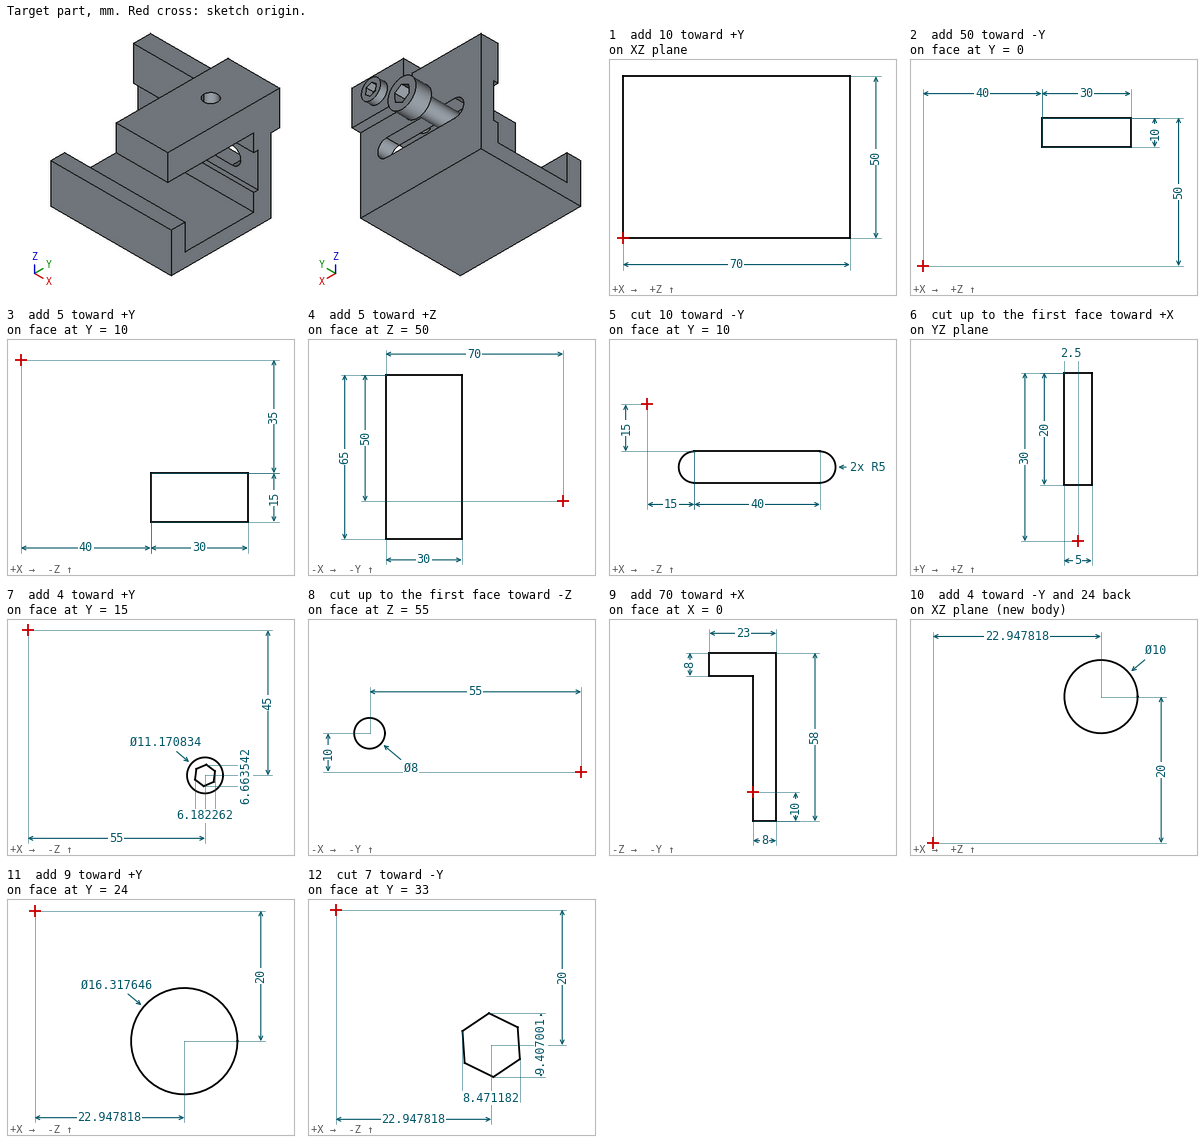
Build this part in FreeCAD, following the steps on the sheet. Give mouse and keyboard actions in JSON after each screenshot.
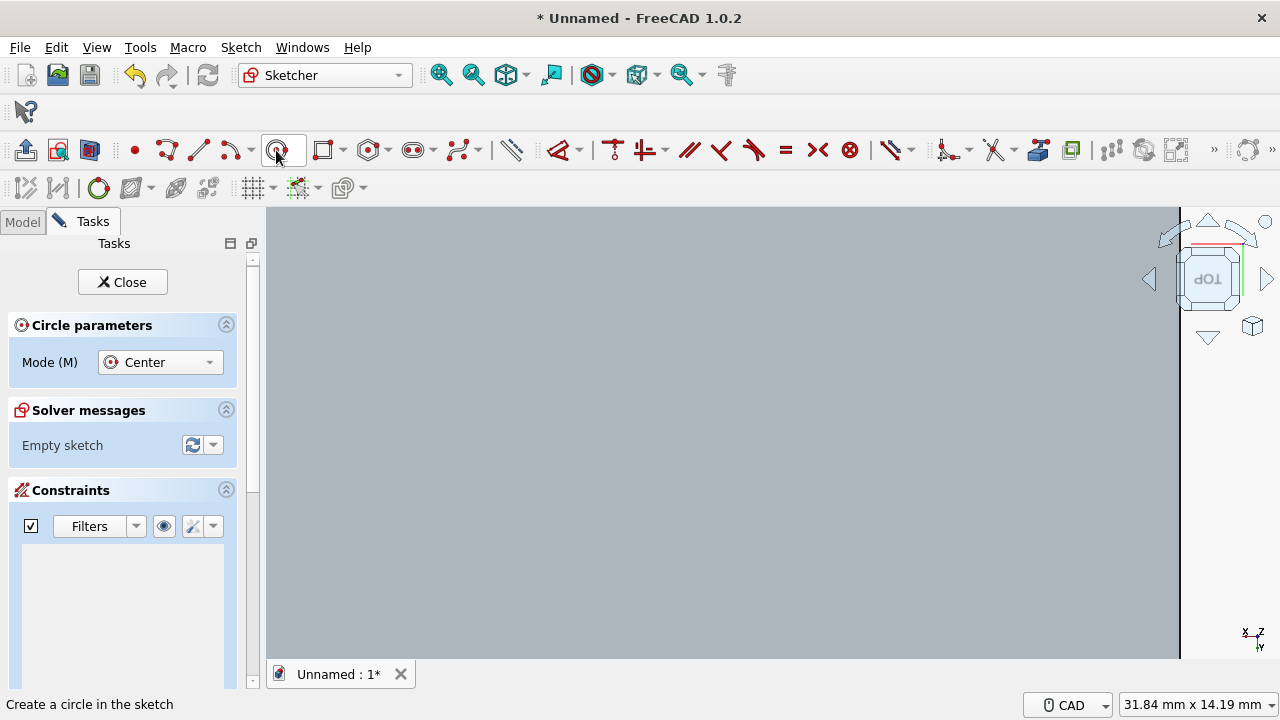
{"action": "left_click", "coordinate": [702, 429]}
{"action": "left_click", "coordinate": [792, 339]}
{"action": "key", "text": "Escape"}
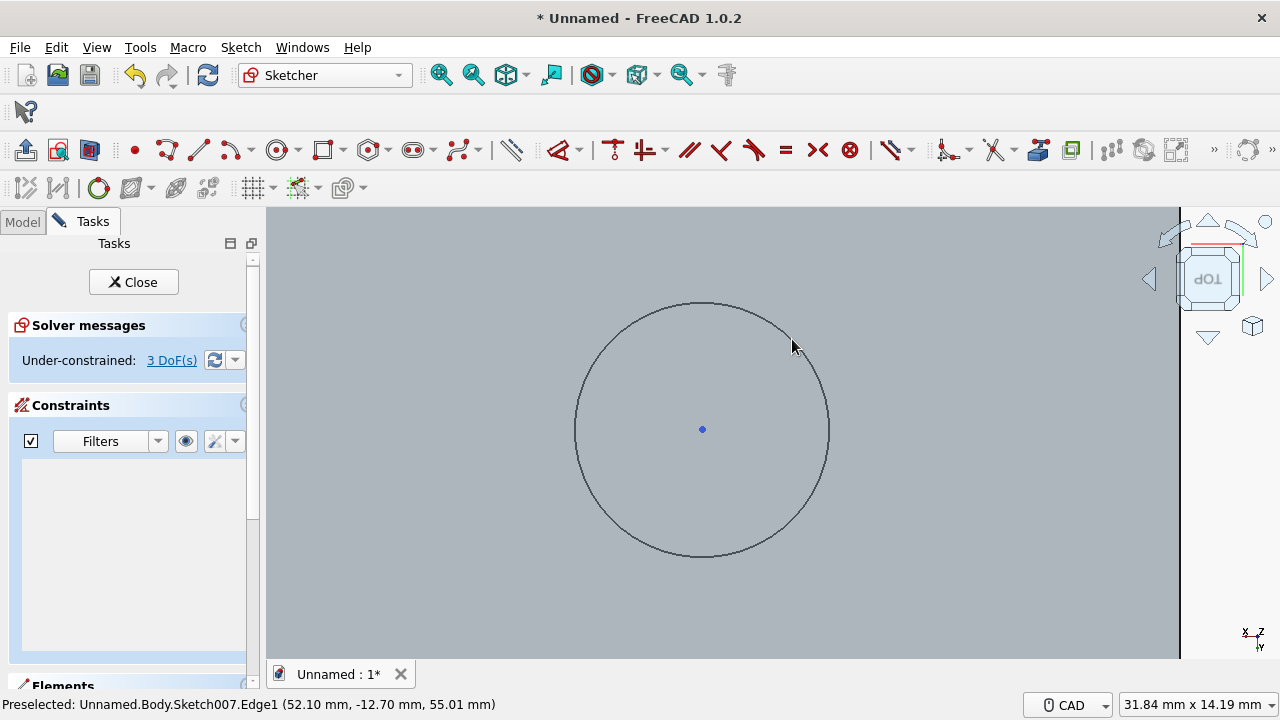
{"action": "left_click", "coordinate": [558, 150]}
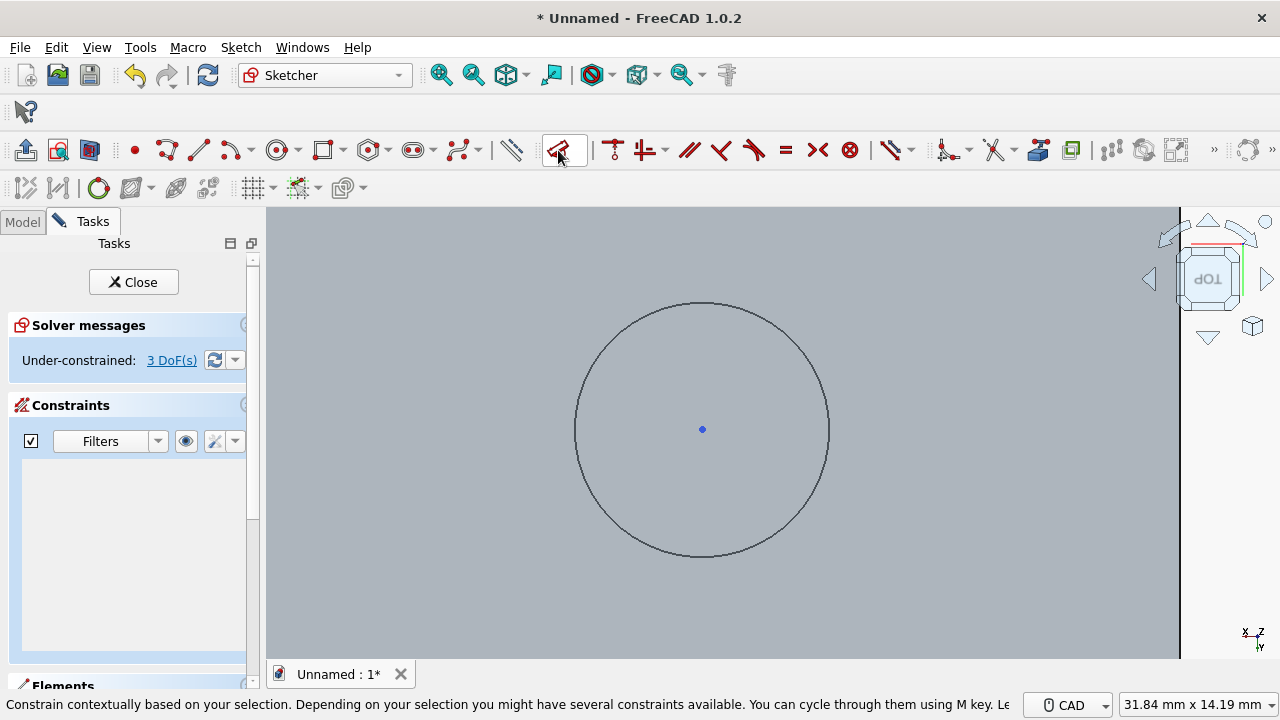
{"action": "left_click", "coordinate": [792, 340]}
{"action": "left_click", "coordinate": [815, 317]}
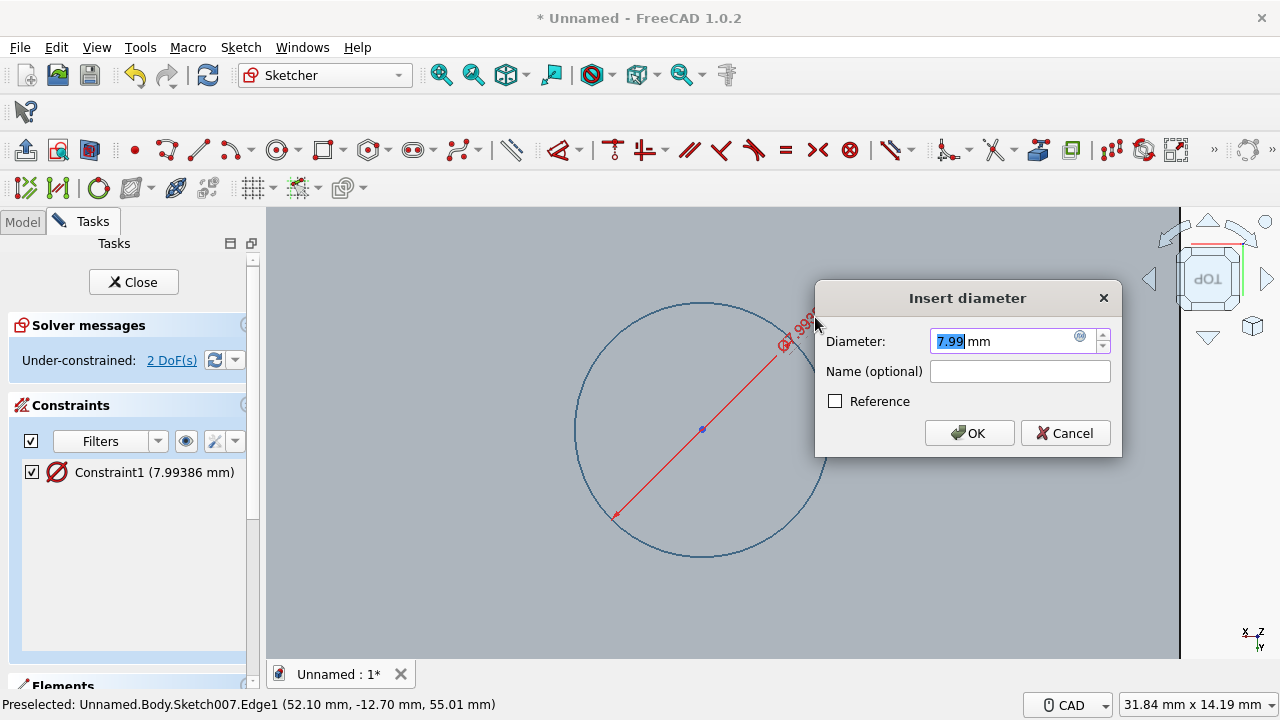
{"action": "type", "text": "8"}
{"action": "key", "text": "Return"}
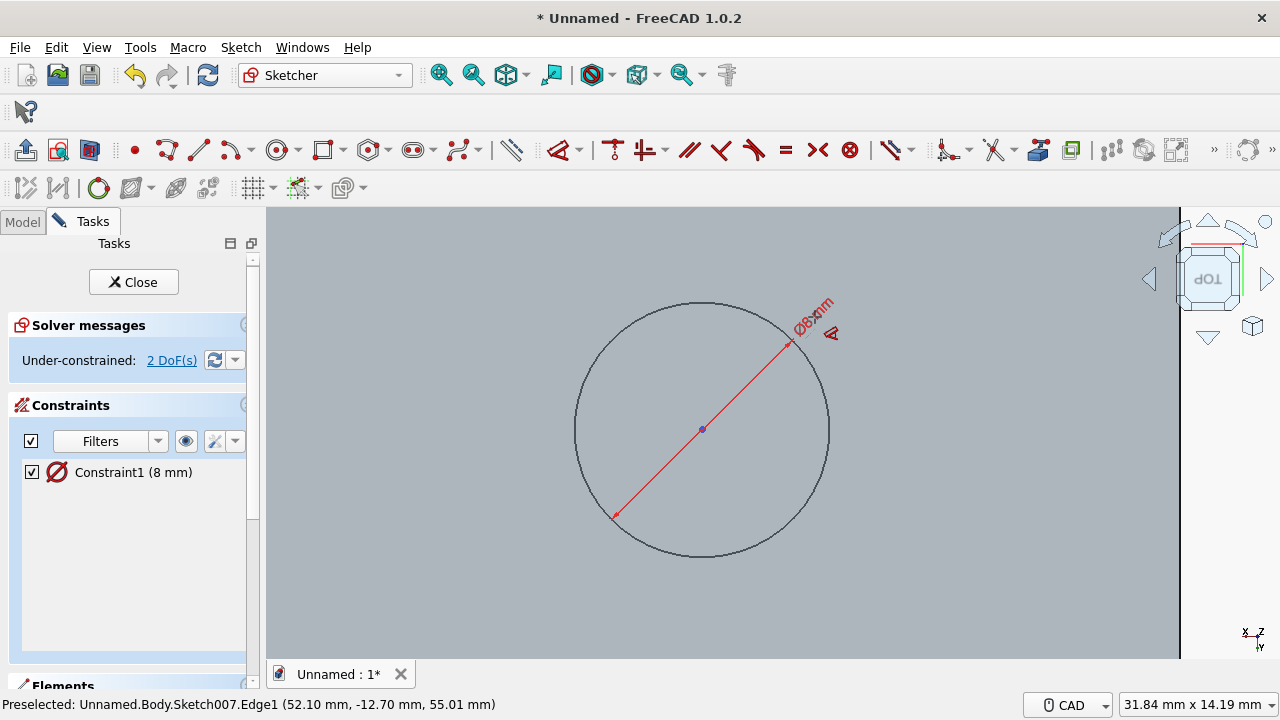
{"action": "left_click", "coordinate": [702, 430]}
{"action": "left_click", "coordinate": [909, 396]}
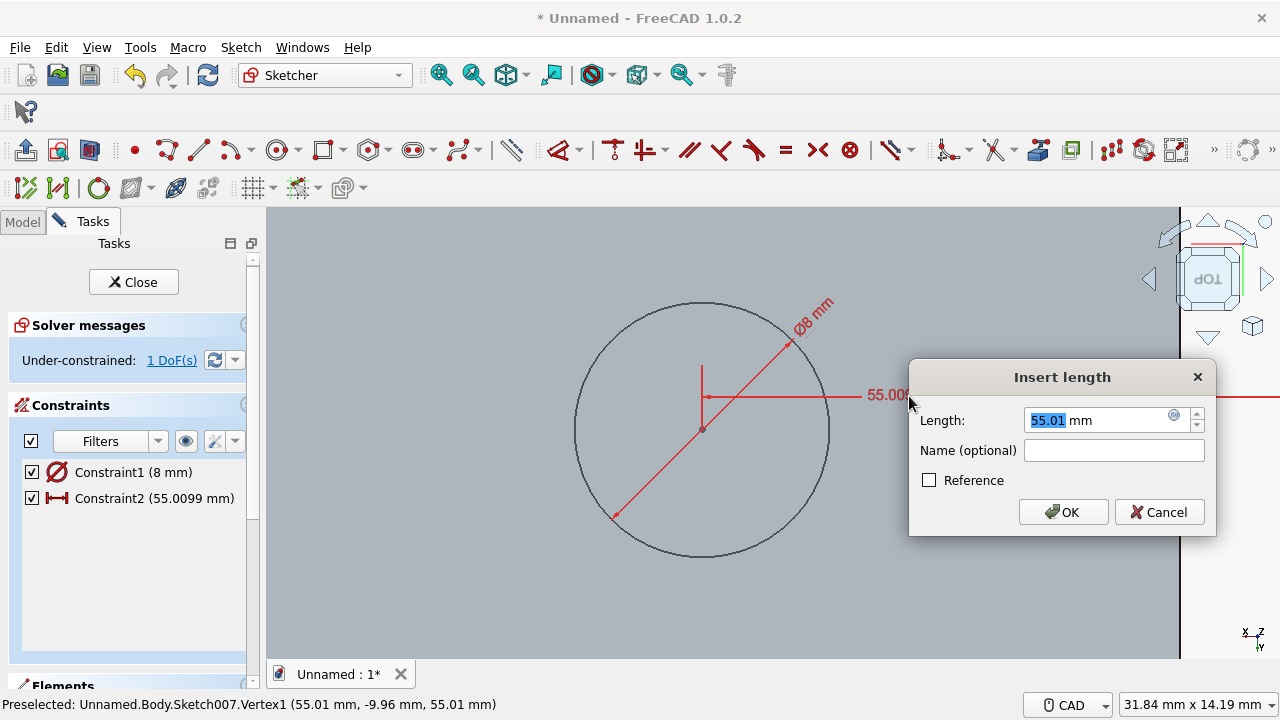
{"action": "type", "text": "55"}
{"action": "key", "text": "Return"}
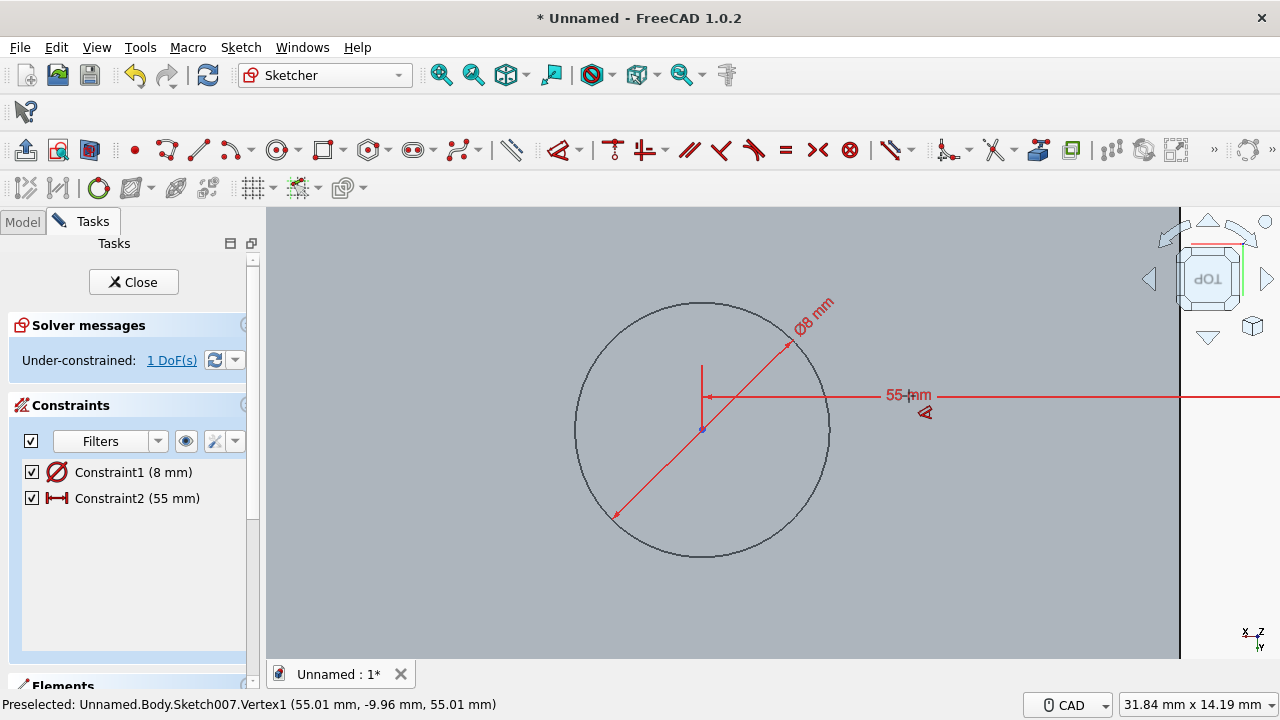
{"action": "left_click", "coordinate": [702, 430]}
{"action": "left_click", "coordinate": [668, 530]}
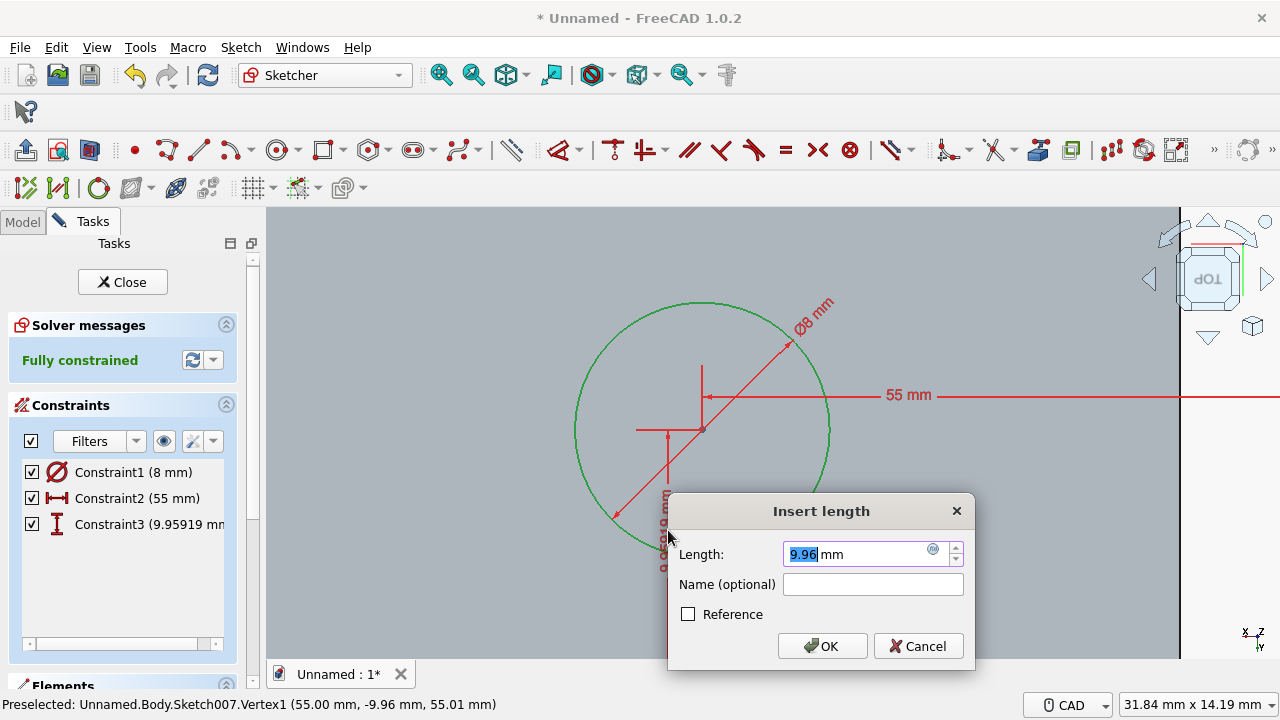
{"action": "type", "text": "10"}
{"action": "key", "text": "Return"}
{"action": "key", "text": "Escape"}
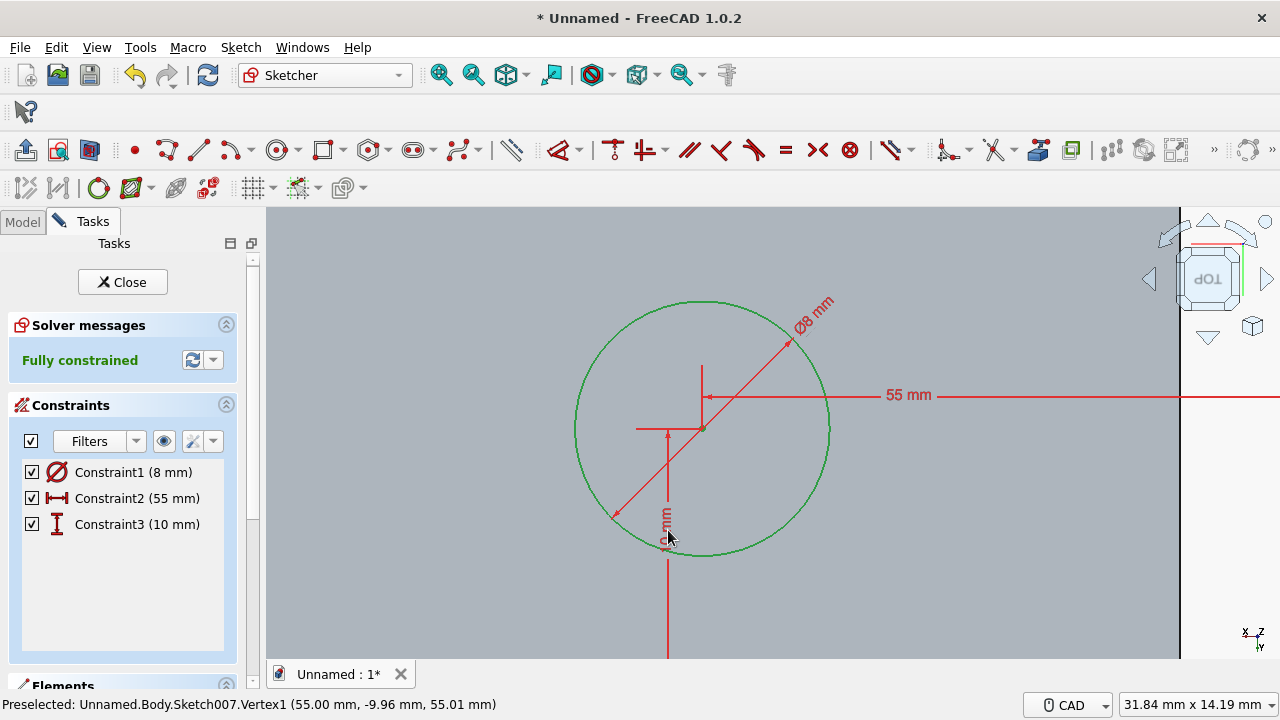
{"action": "left_click", "coordinate": [123, 282]}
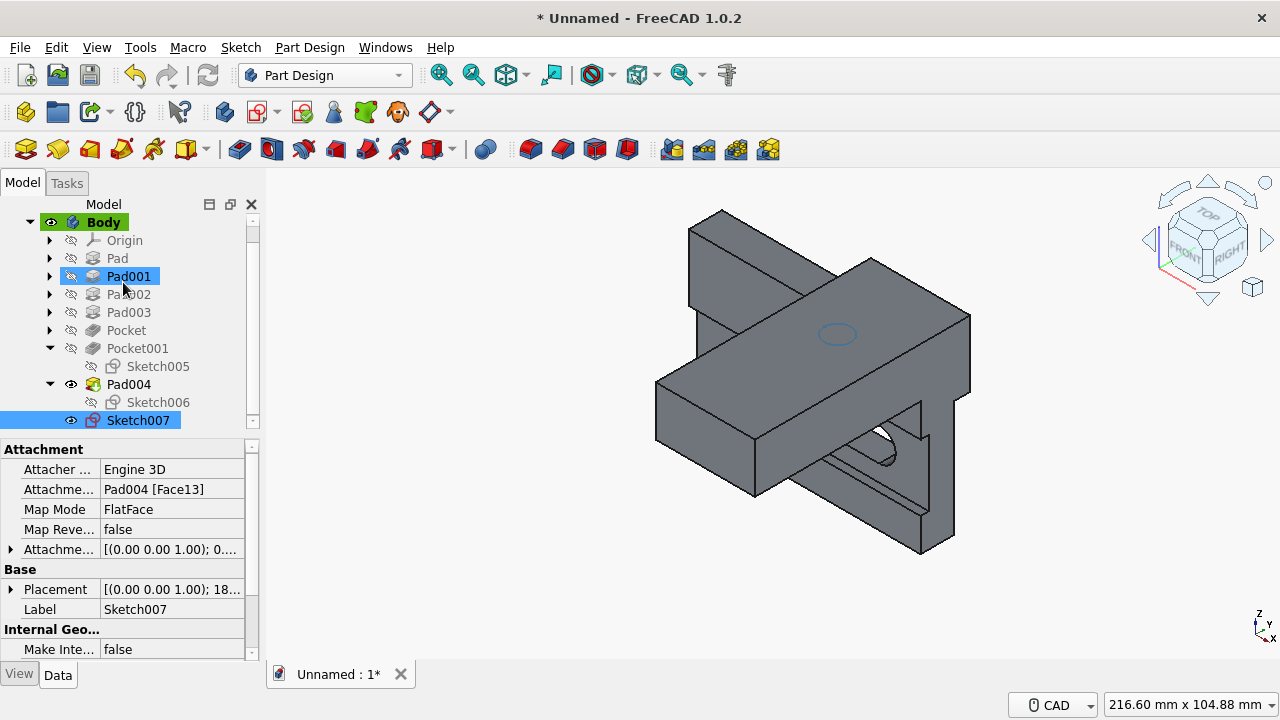
{"action": "left_click", "coordinate": [240, 150]}